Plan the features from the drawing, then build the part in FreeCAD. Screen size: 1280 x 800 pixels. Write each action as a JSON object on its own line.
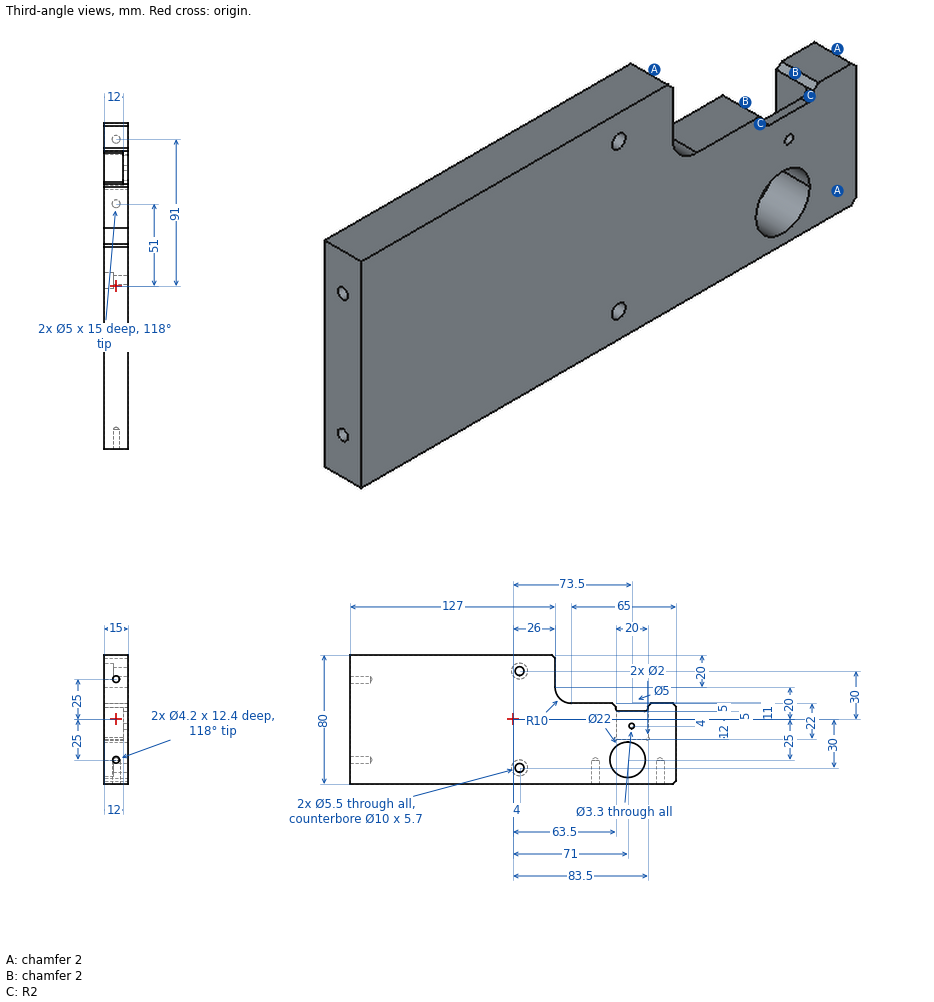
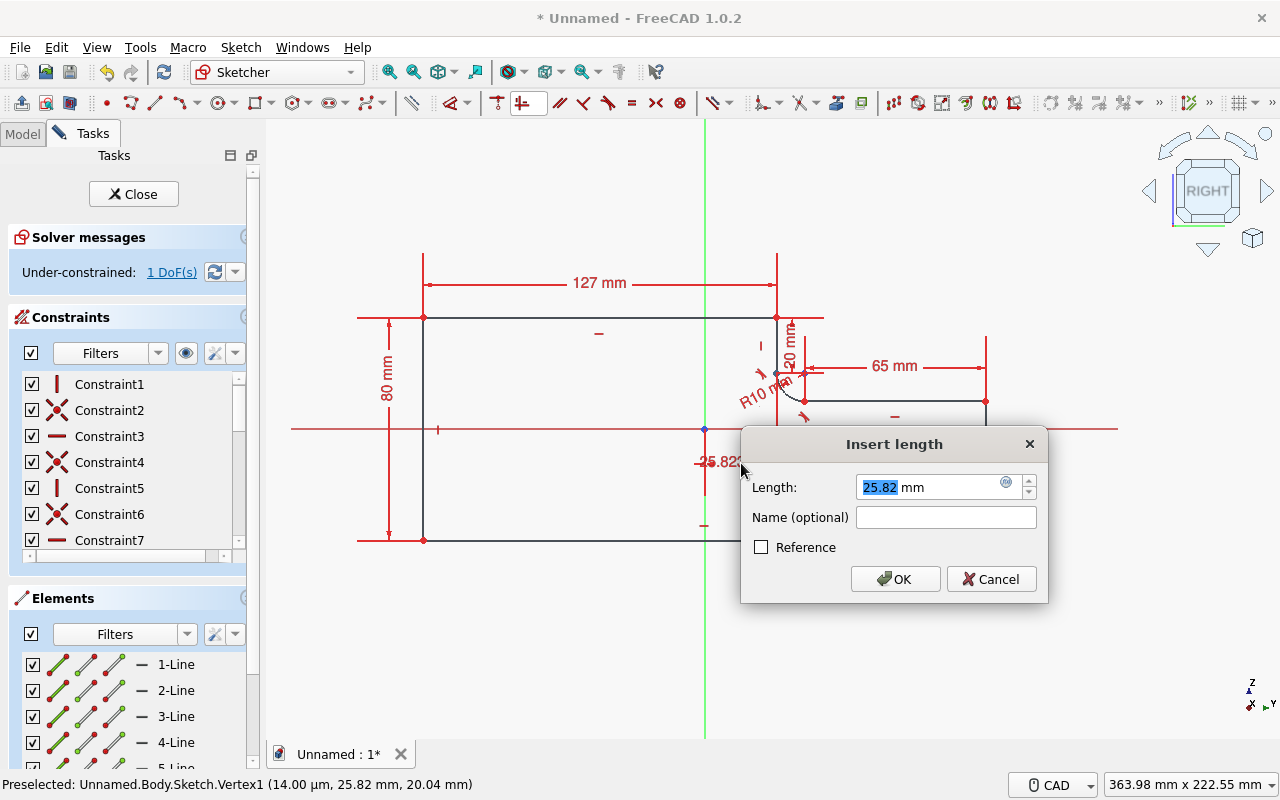
{"action": "type", "text": "26"}
{"action": "key", "text": "Return"}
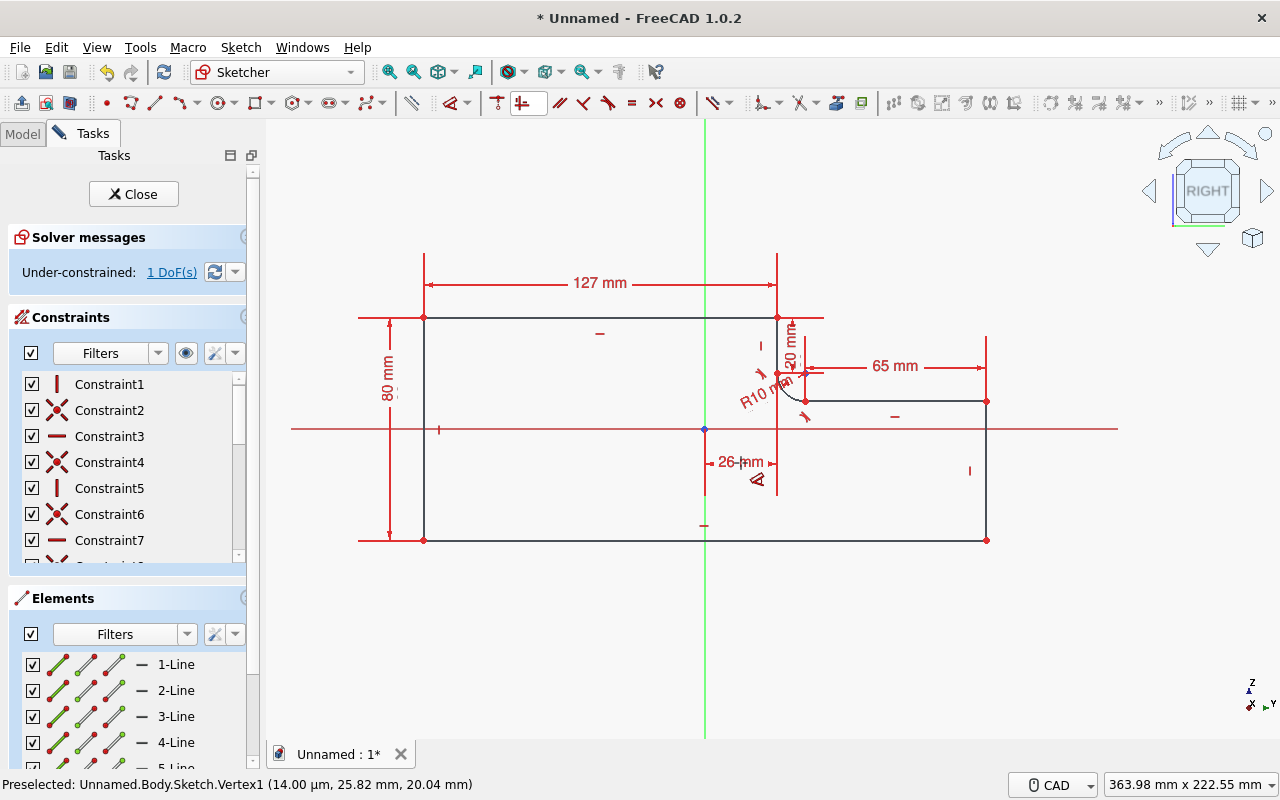
{"action": "left_click", "coordinate": [777, 373]}
{"action": "left_click", "coordinate": [671, 401]}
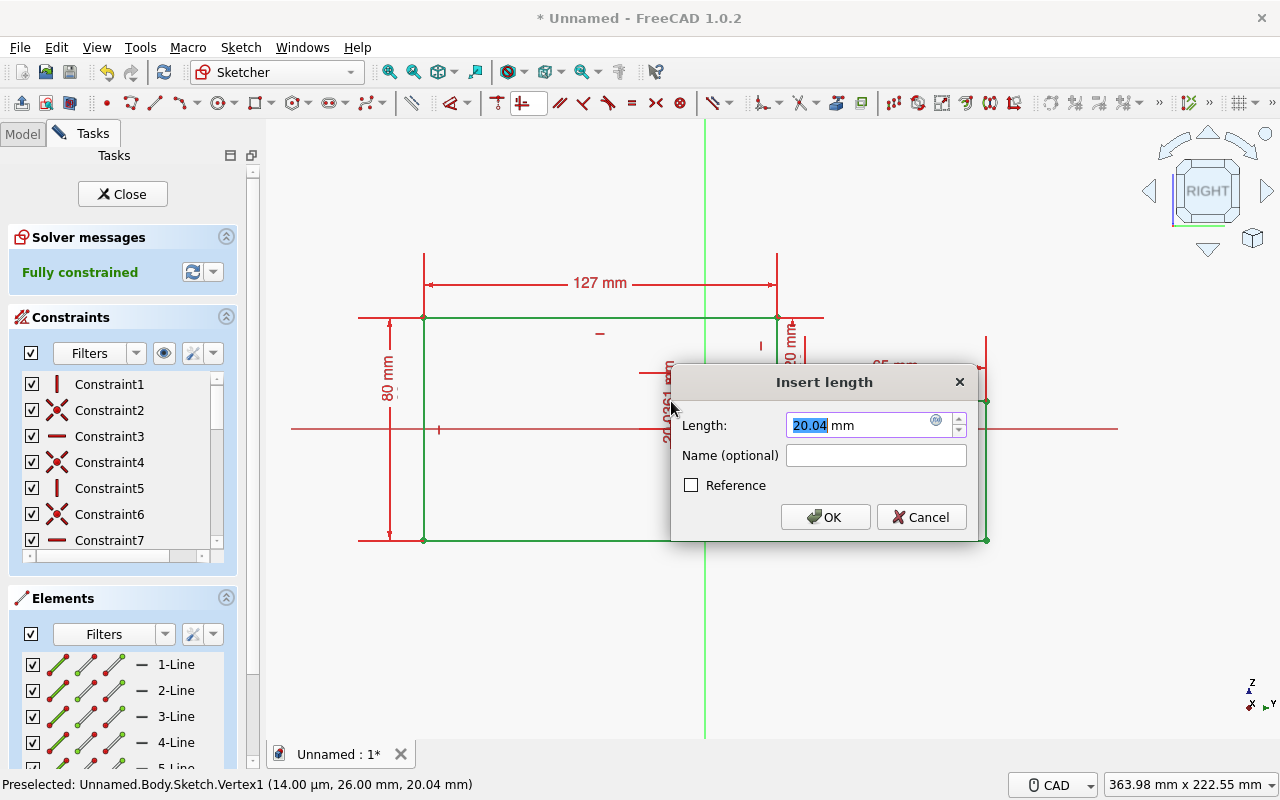
{"action": "type", "text": "20"}
{"action": "key", "text": "Return"}
{"action": "key", "text": "Escape"}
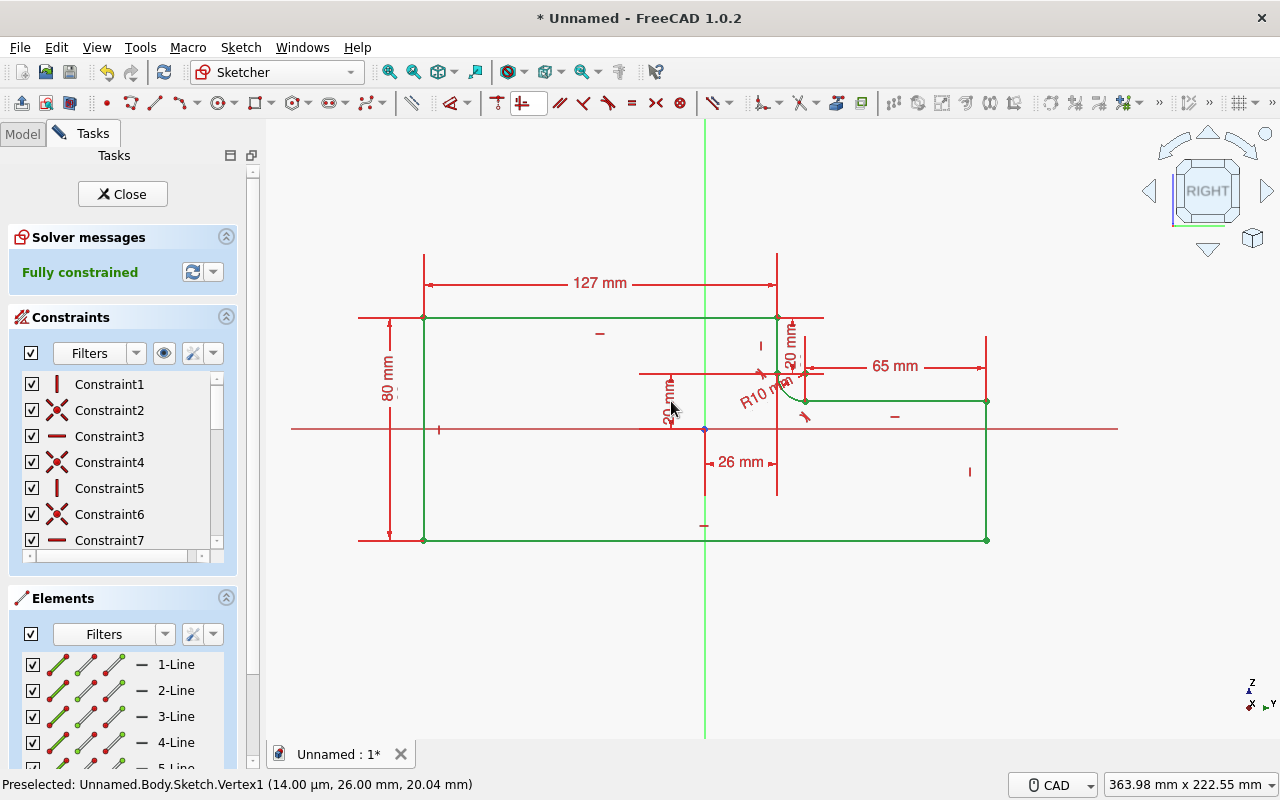
{"action": "left_click", "coordinate": [123, 194]}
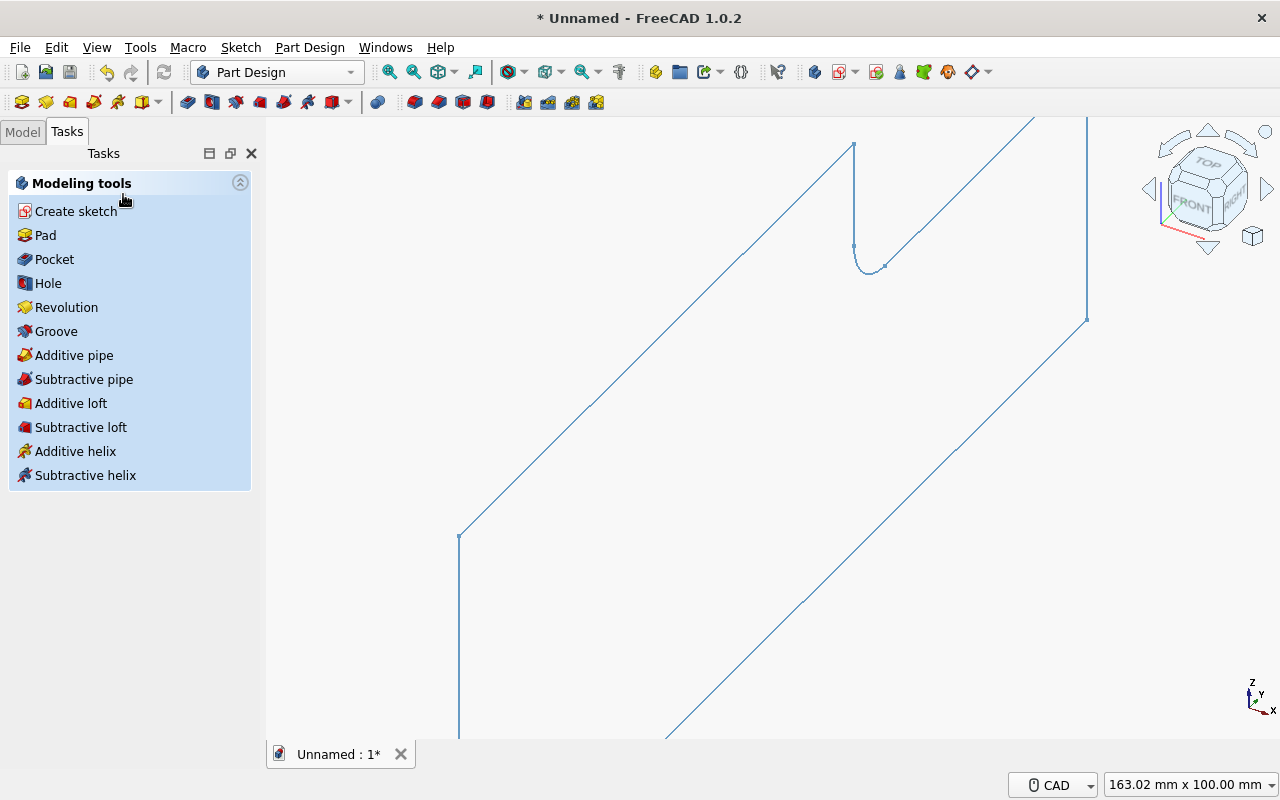
{"action": "left_click", "coordinate": [22, 102]}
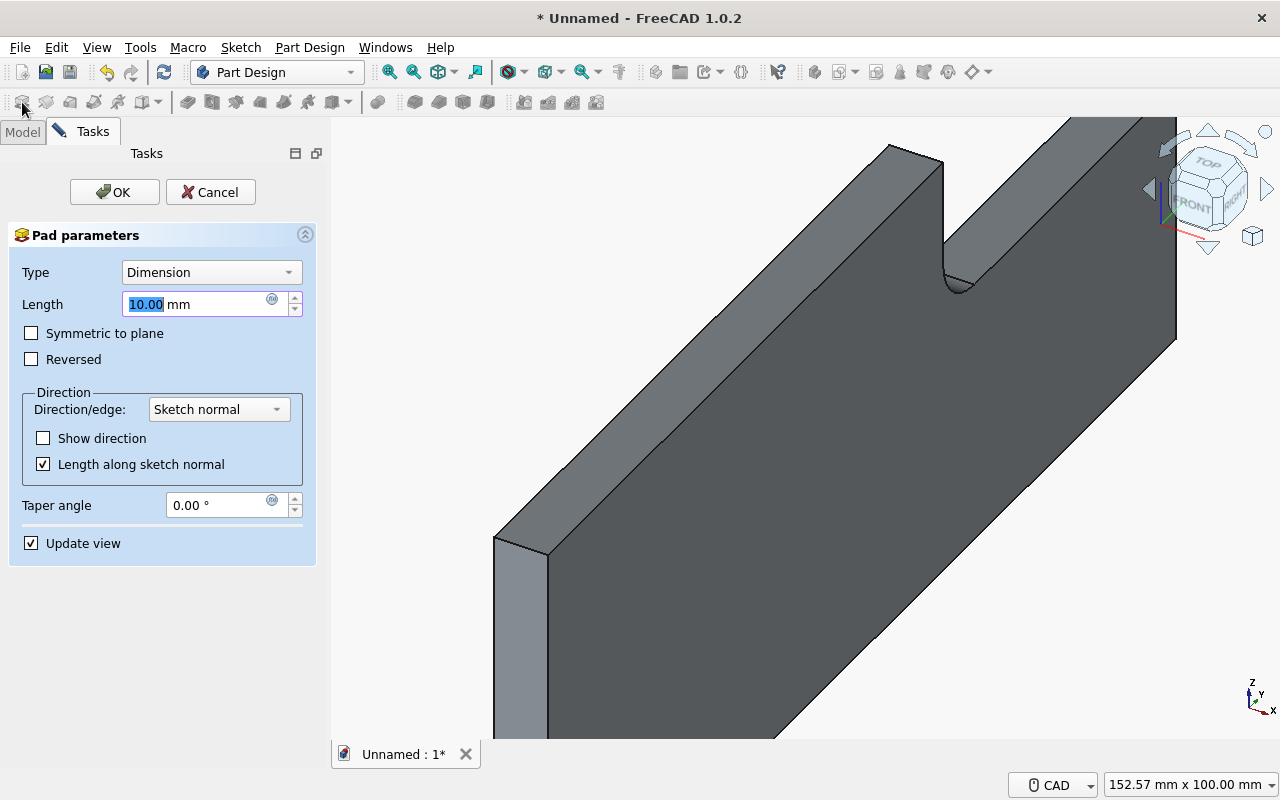
{"action": "type", "text": "15"}
{"action": "key", "text": "Tab"}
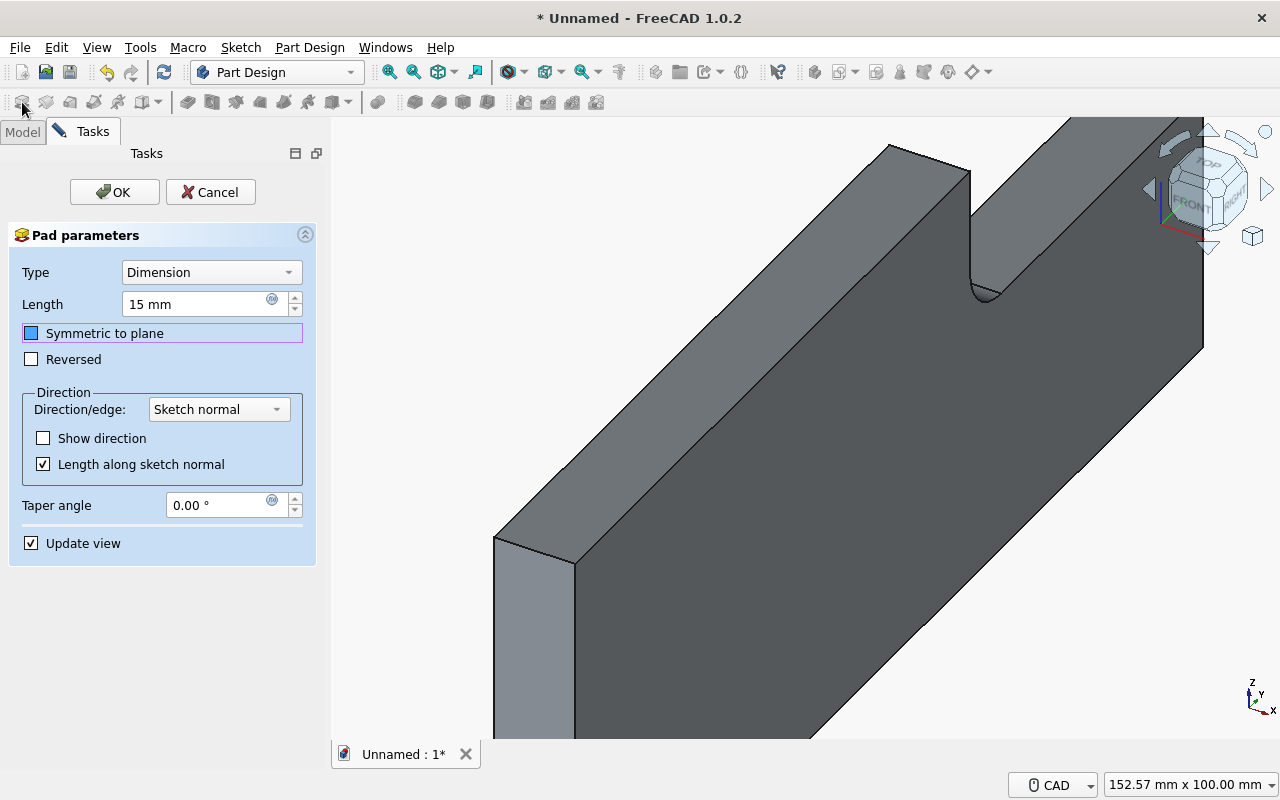
{"action": "left_click", "coordinate": [30, 333]}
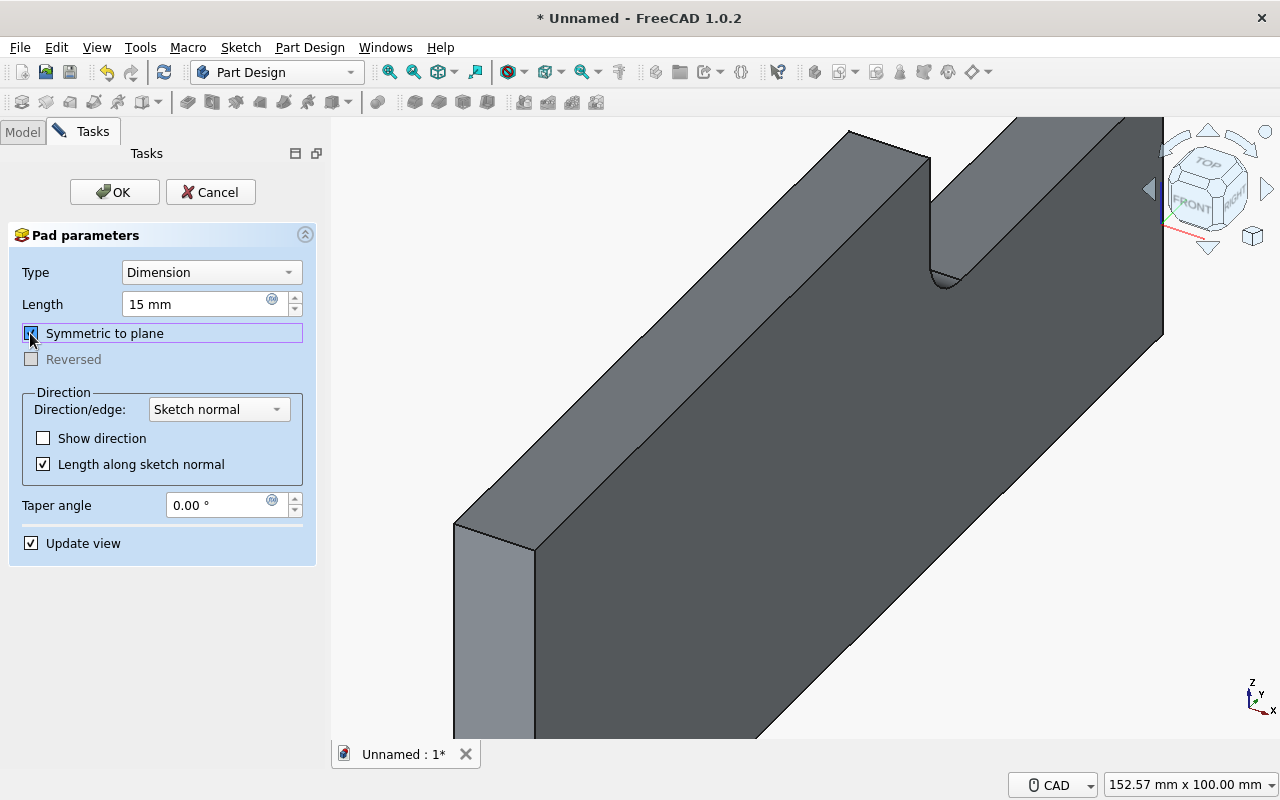
{"action": "left_click", "coordinate": [115, 192]}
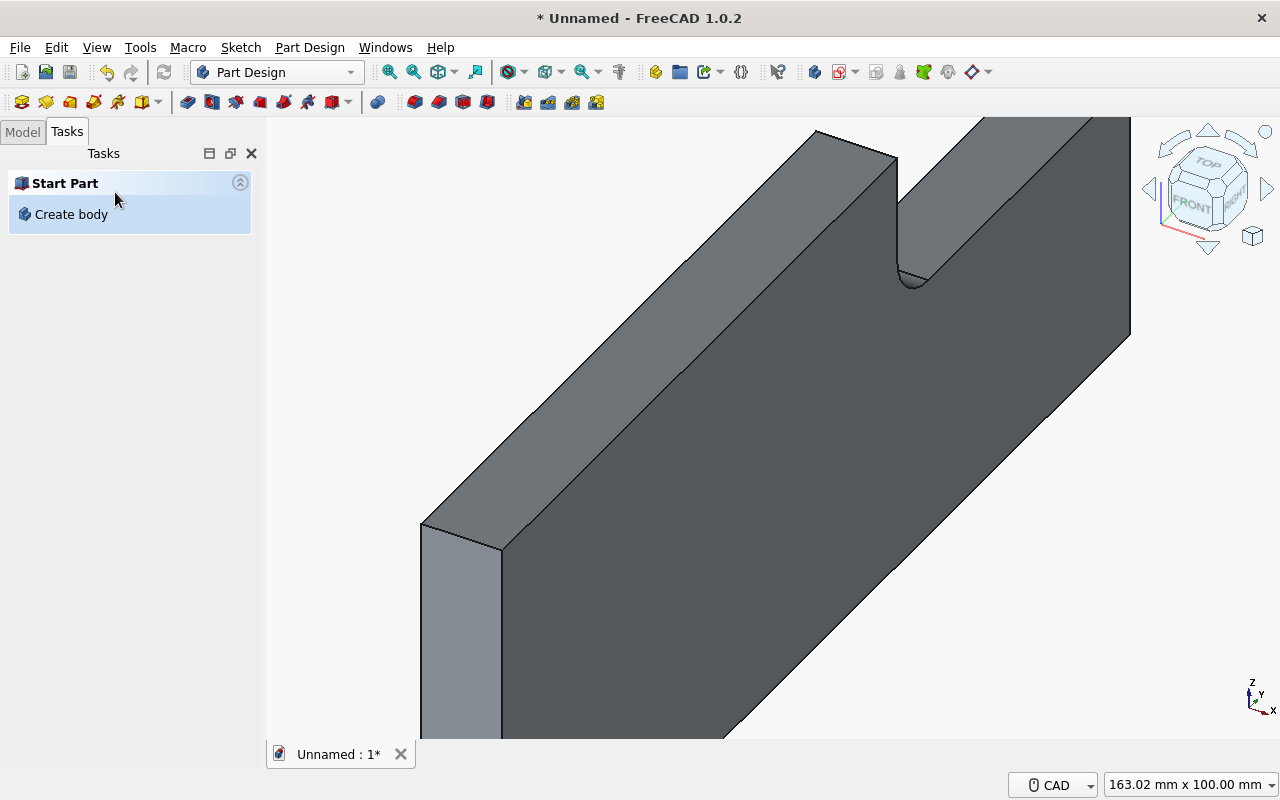
{"action": "left_click", "coordinate": [390, 72]}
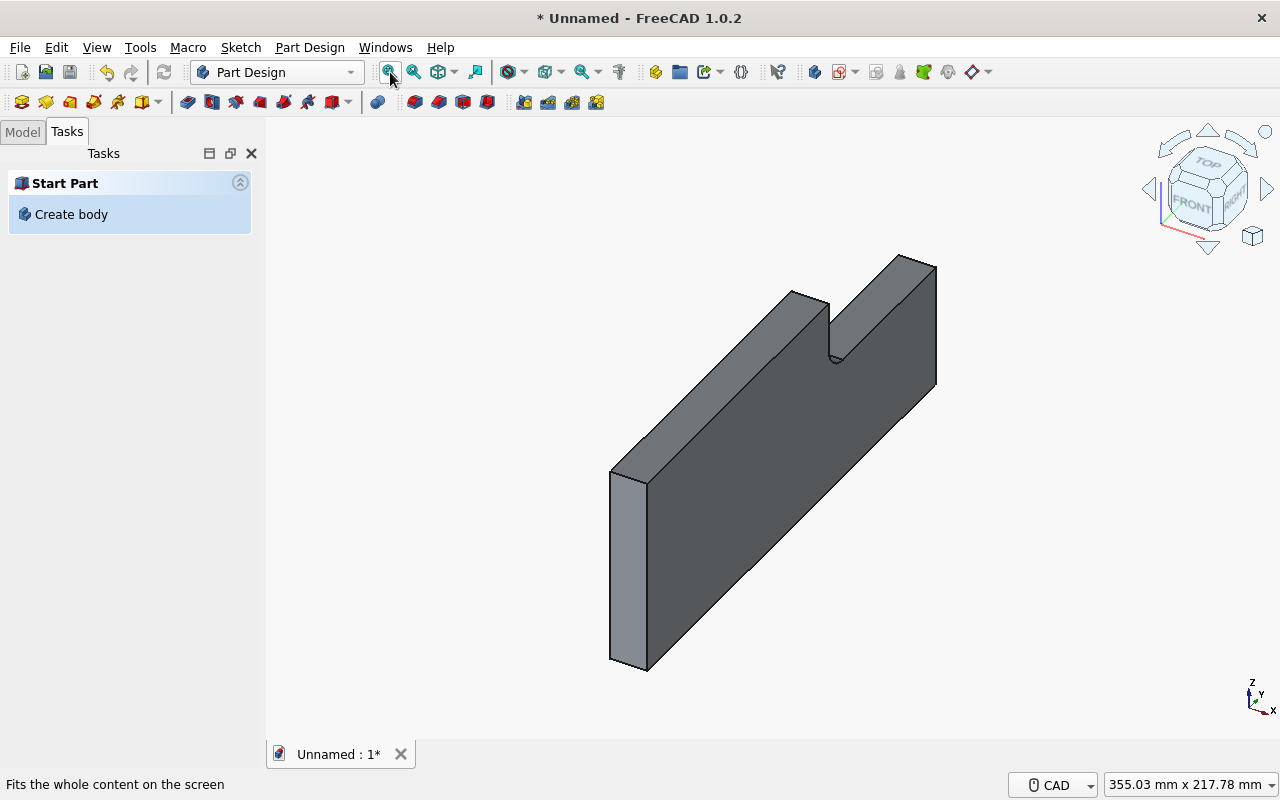
{"action": "key", "text": "6"}